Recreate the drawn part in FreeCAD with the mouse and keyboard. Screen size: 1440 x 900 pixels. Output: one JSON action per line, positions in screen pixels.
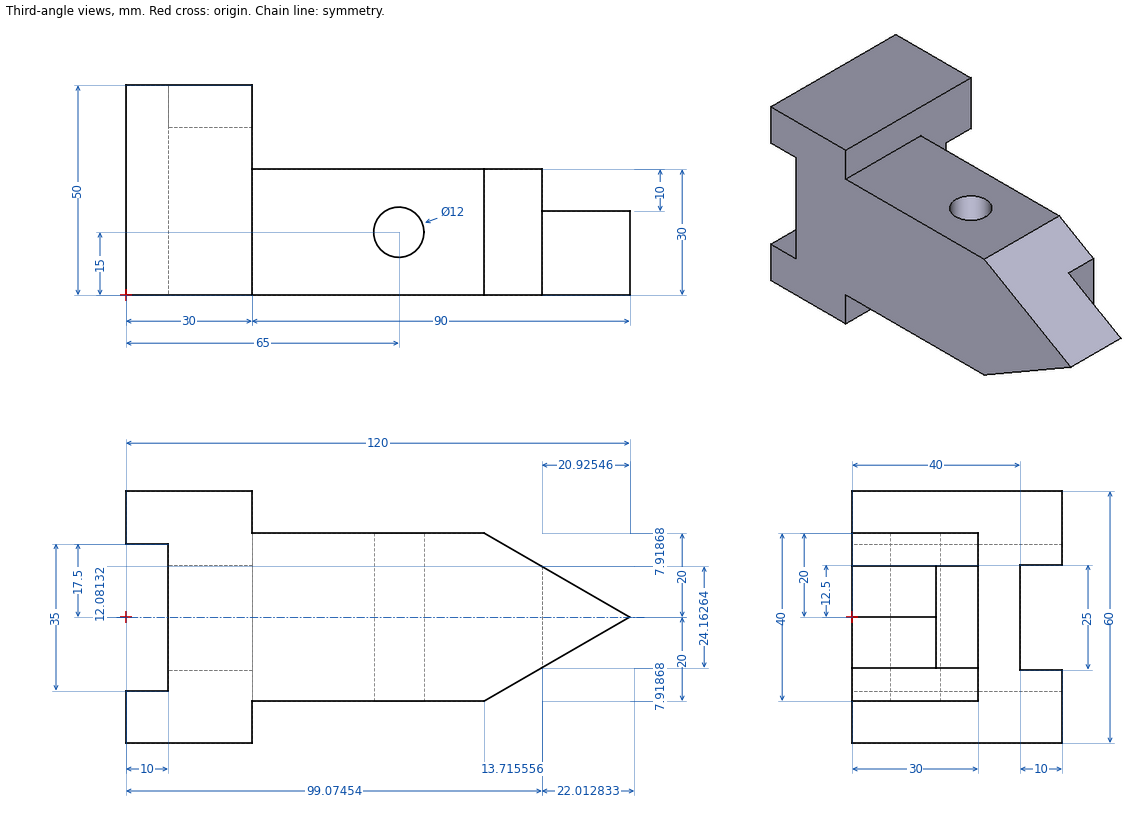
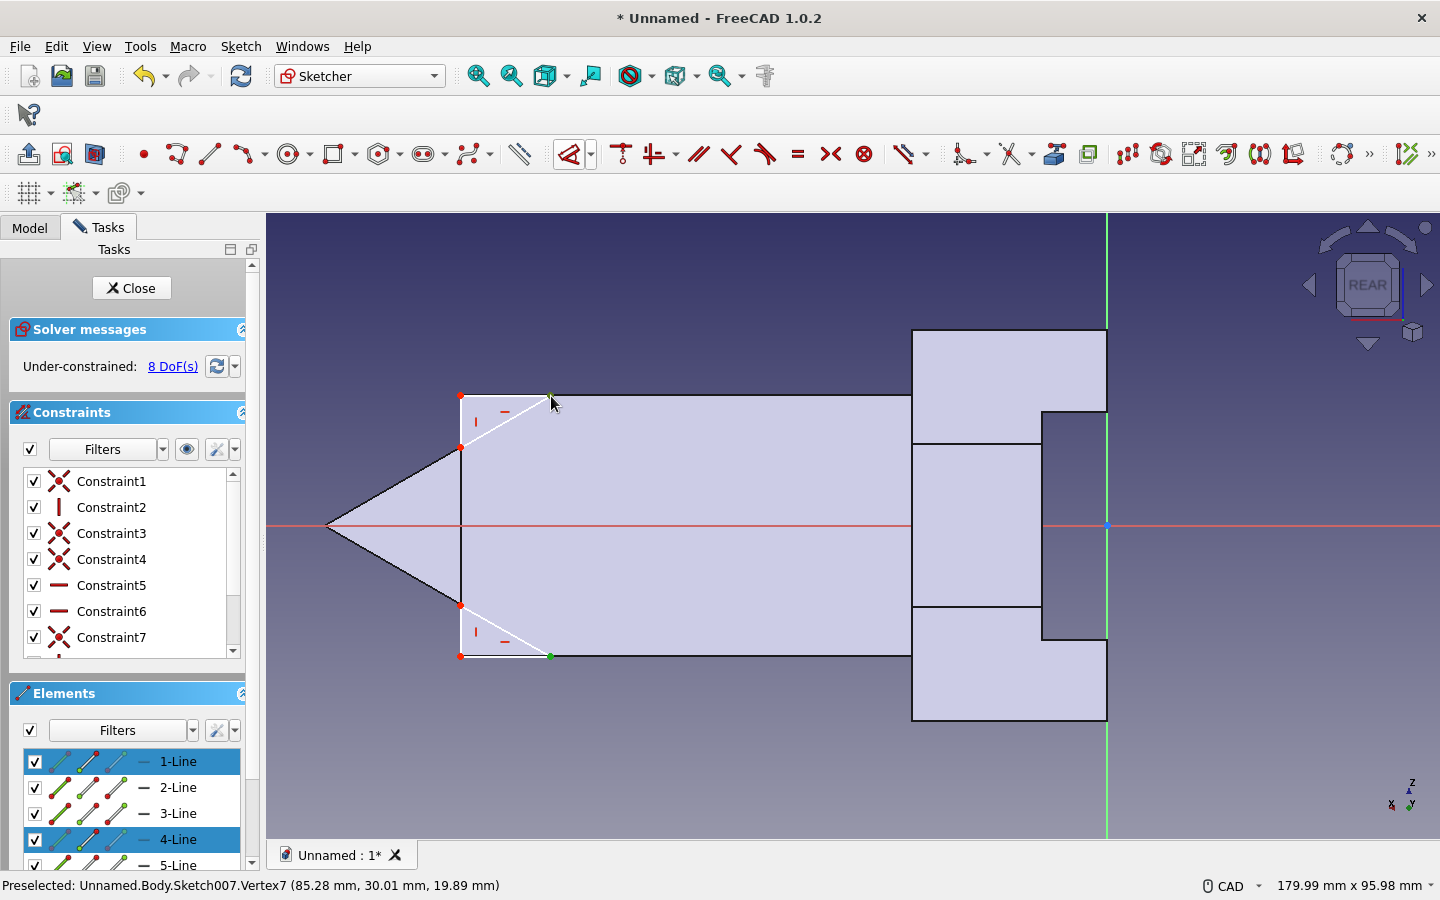
{"action": "left_click", "coordinate": [364, 526]}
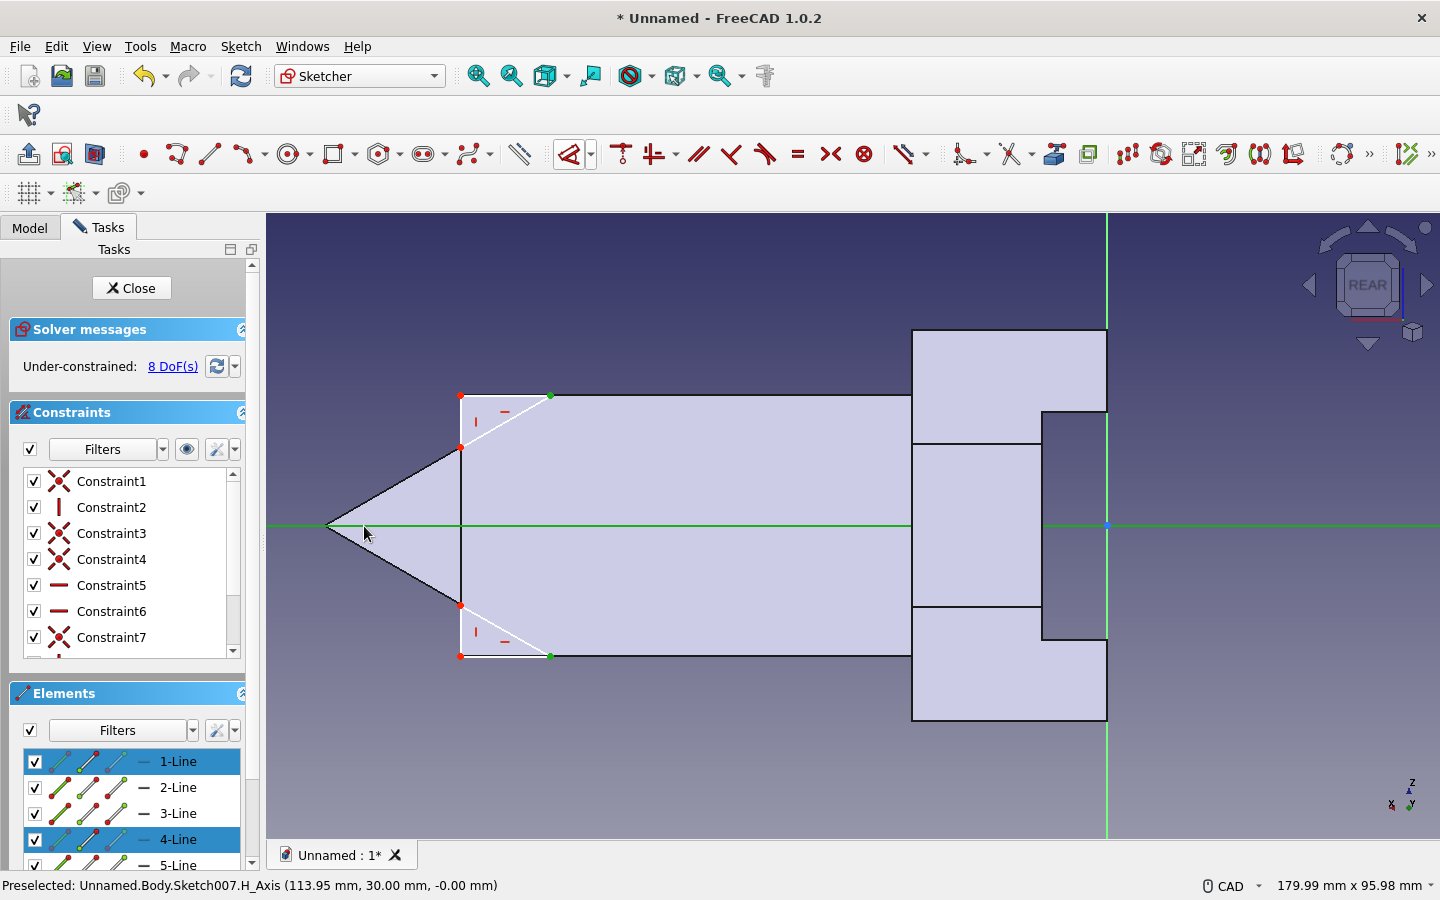
{"action": "left_click", "coordinate": [831, 154]}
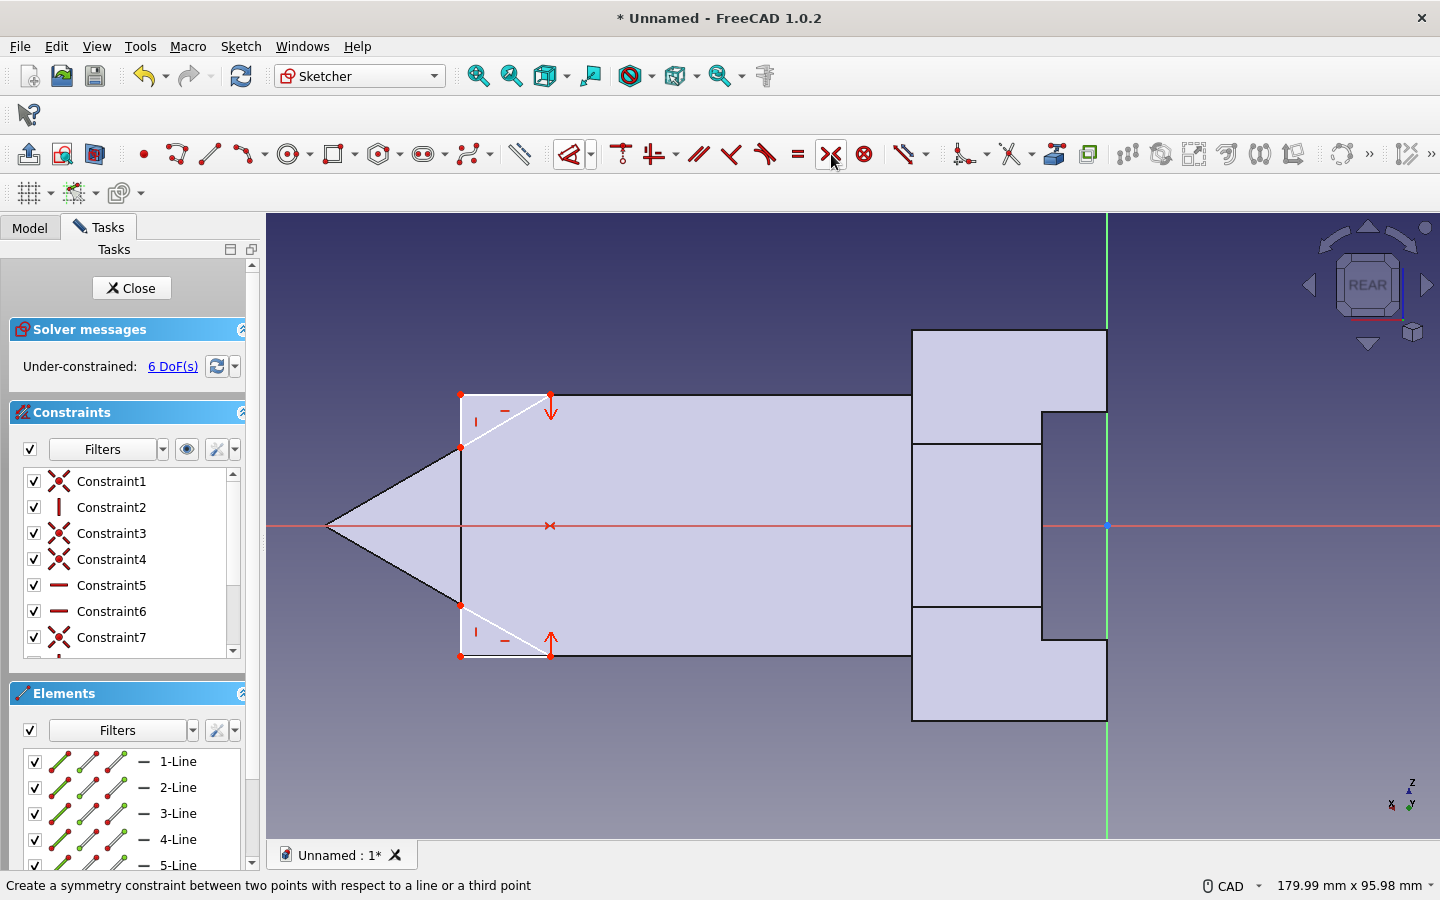
{"action": "left_click", "coordinate": [461, 606]}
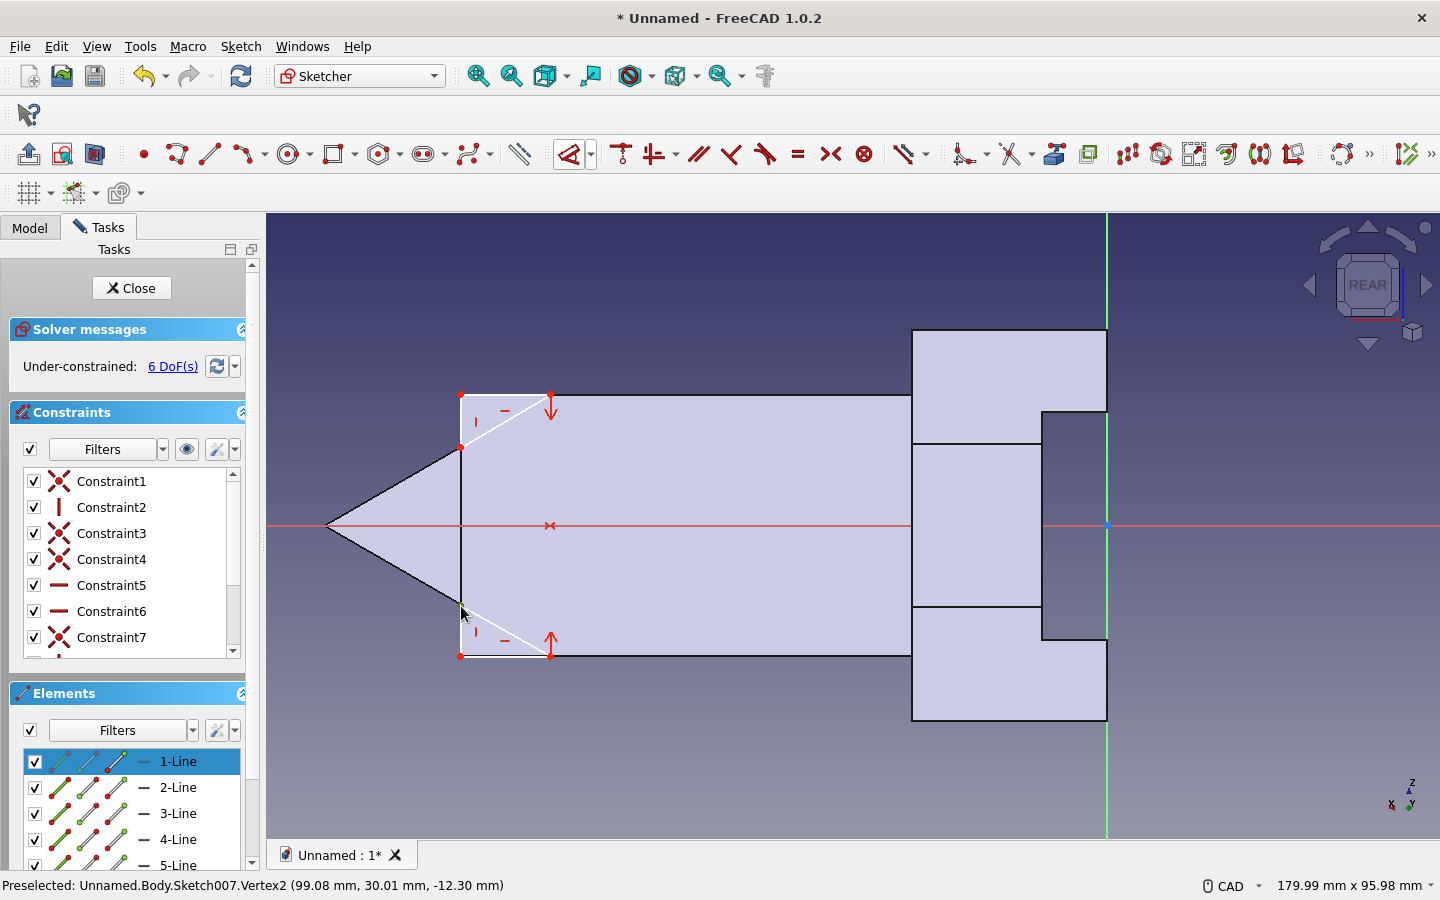
{"action": "left_click", "coordinate": [461, 448]}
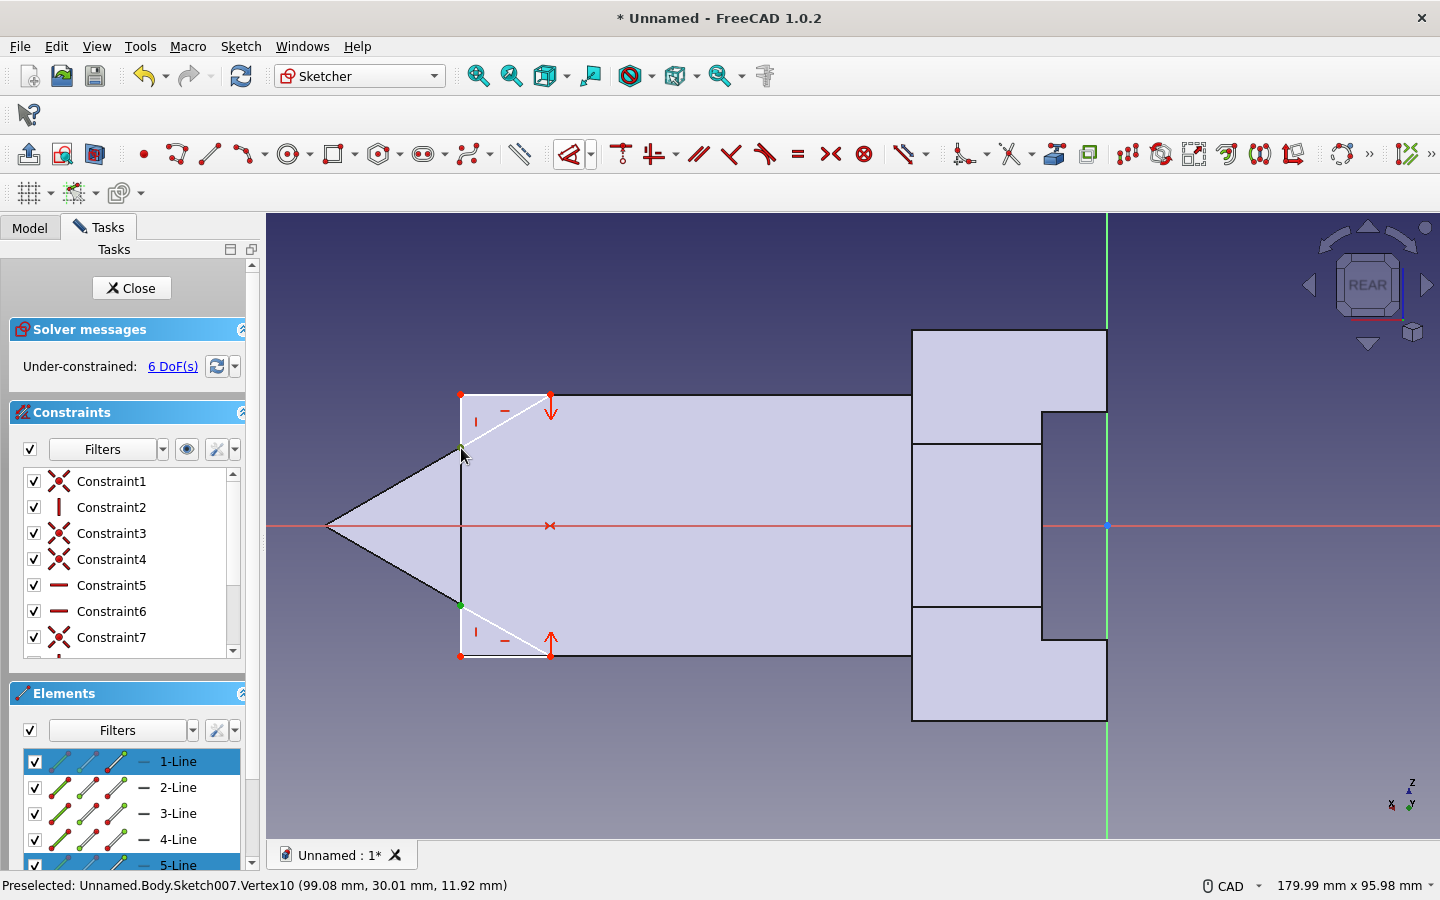
{"action": "left_click", "coordinate": [364, 526]}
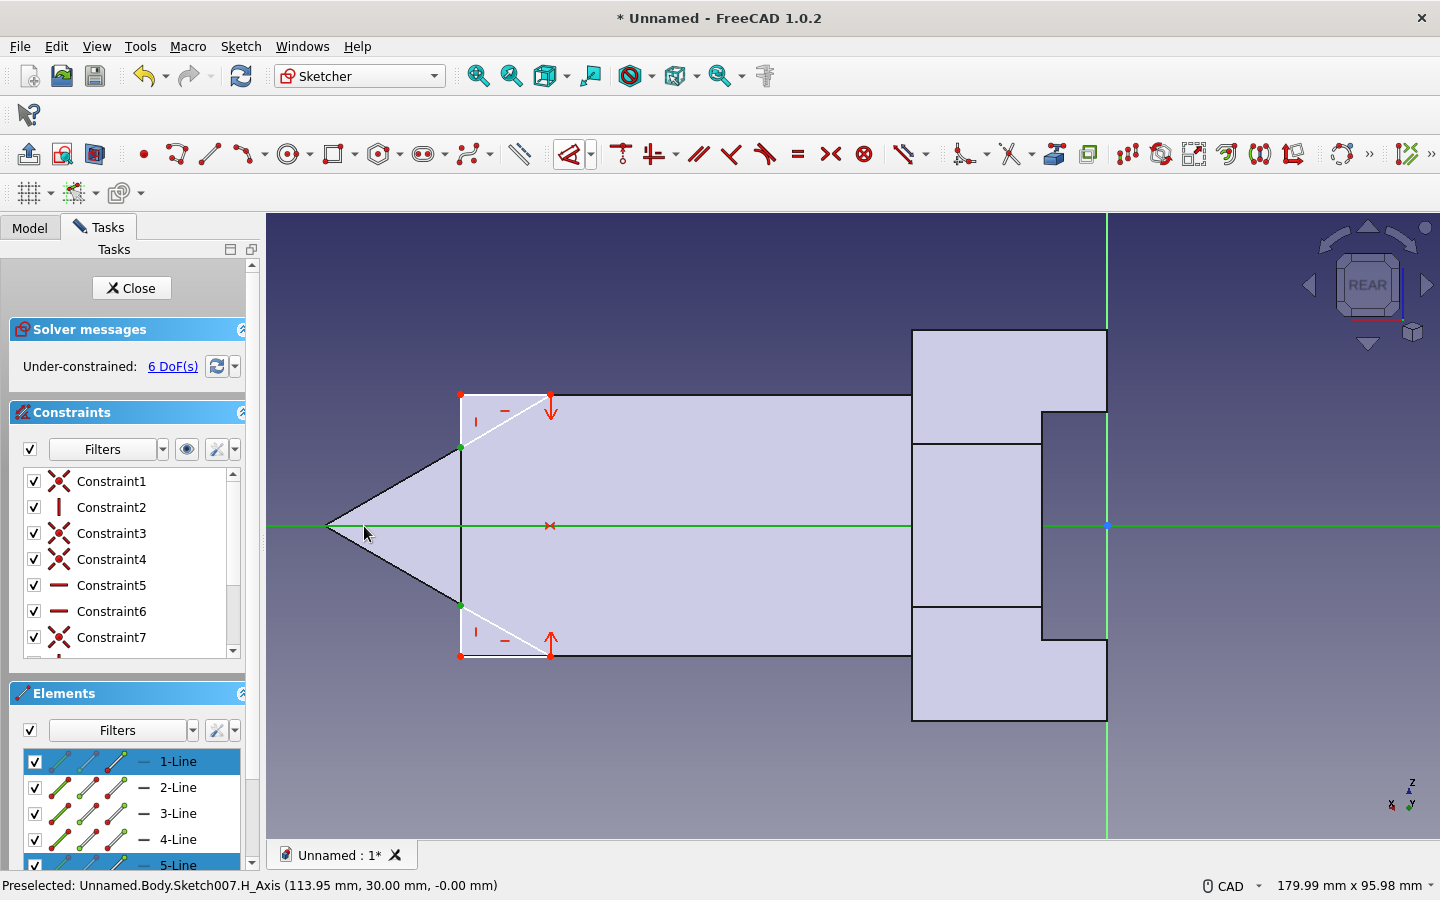
{"action": "key", "text": "s"}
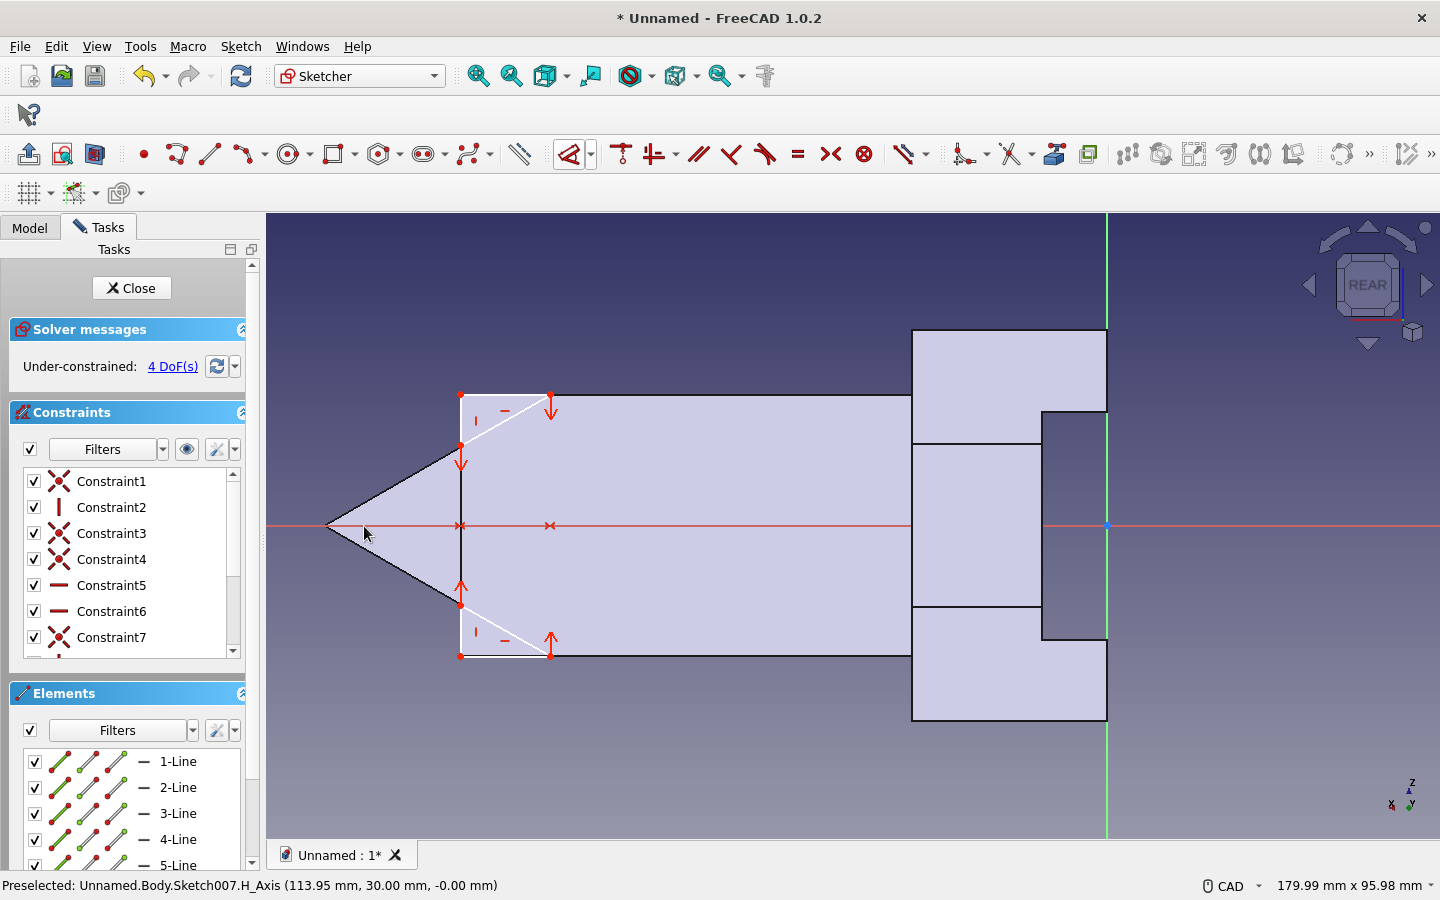
{"action": "left_click", "coordinate": [551, 657]}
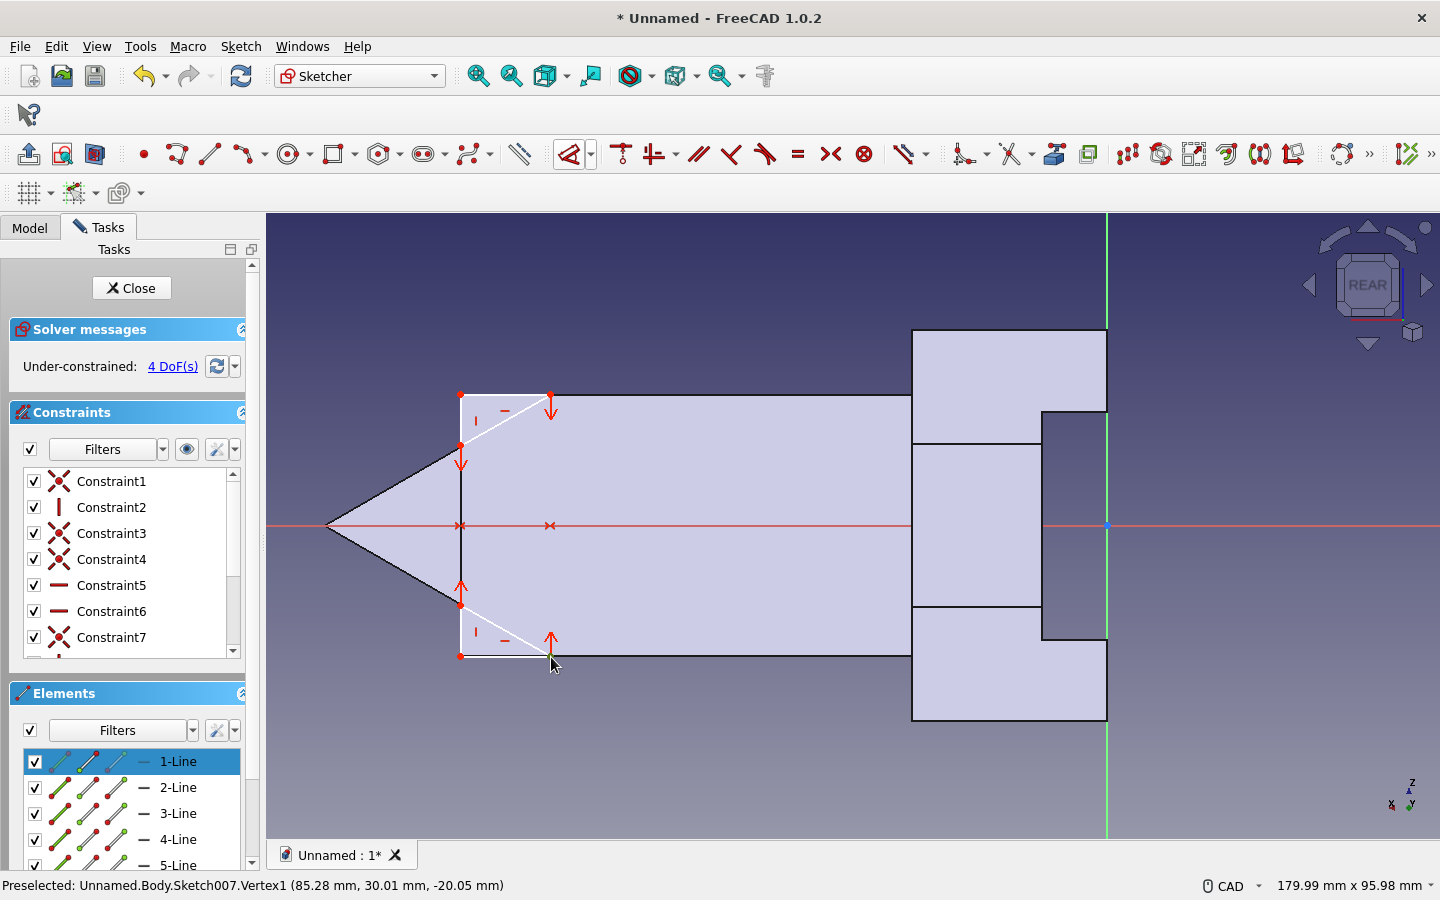
{"action": "left_click", "coordinate": [590, 154]}